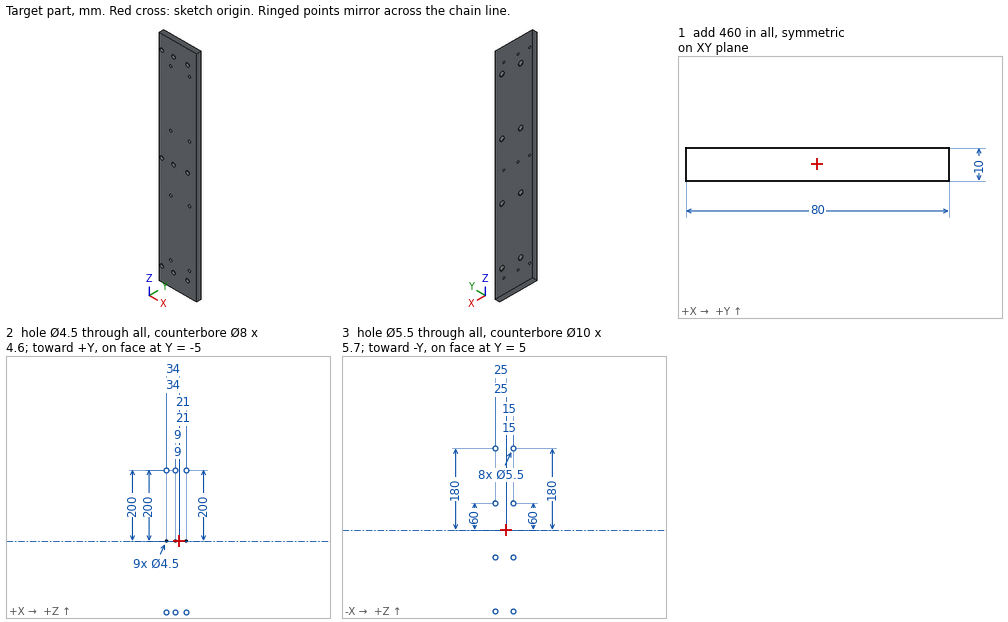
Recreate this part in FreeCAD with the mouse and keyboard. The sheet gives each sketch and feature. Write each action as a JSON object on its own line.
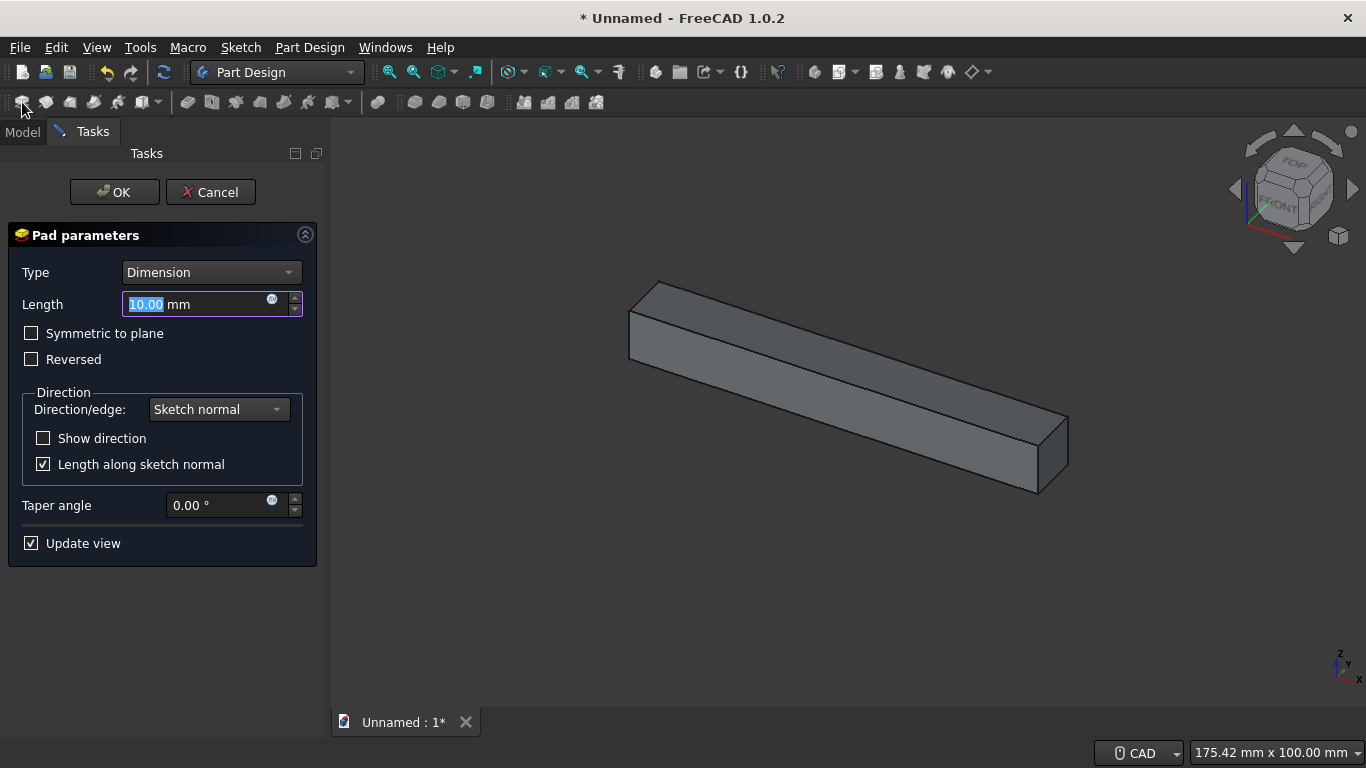
{"action": "type", "text": "460"}
{"action": "key", "text": "Tab"}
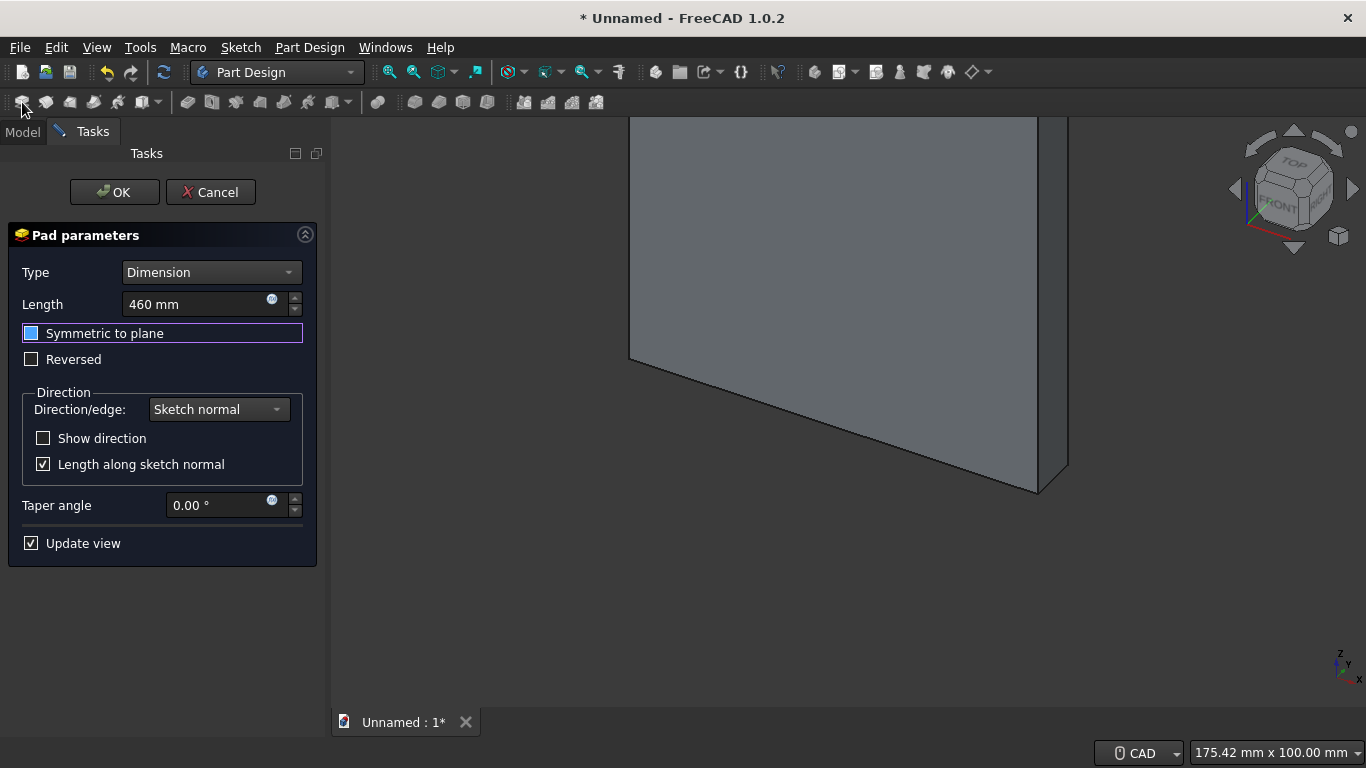
{"action": "left_click", "coordinate": [30, 333]}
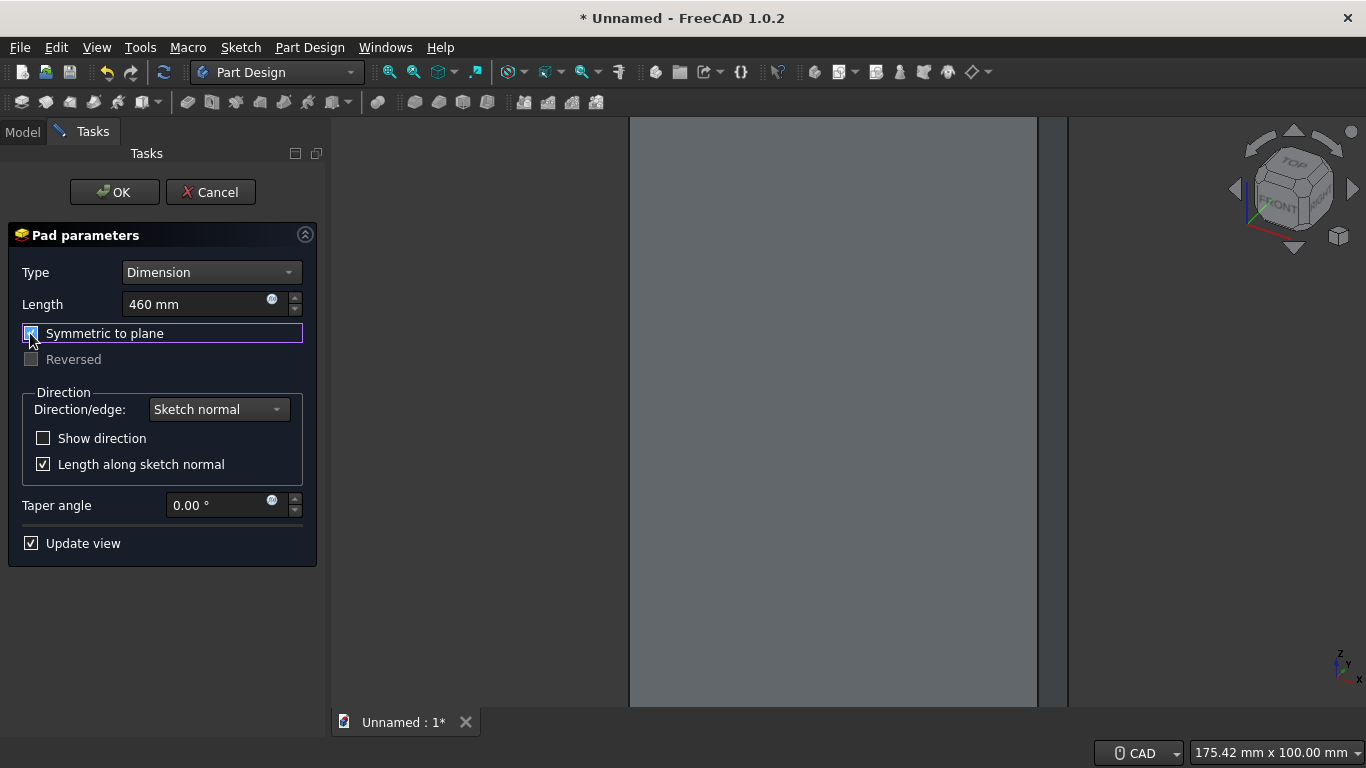
{"action": "left_click", "coordinate": [115, 192]}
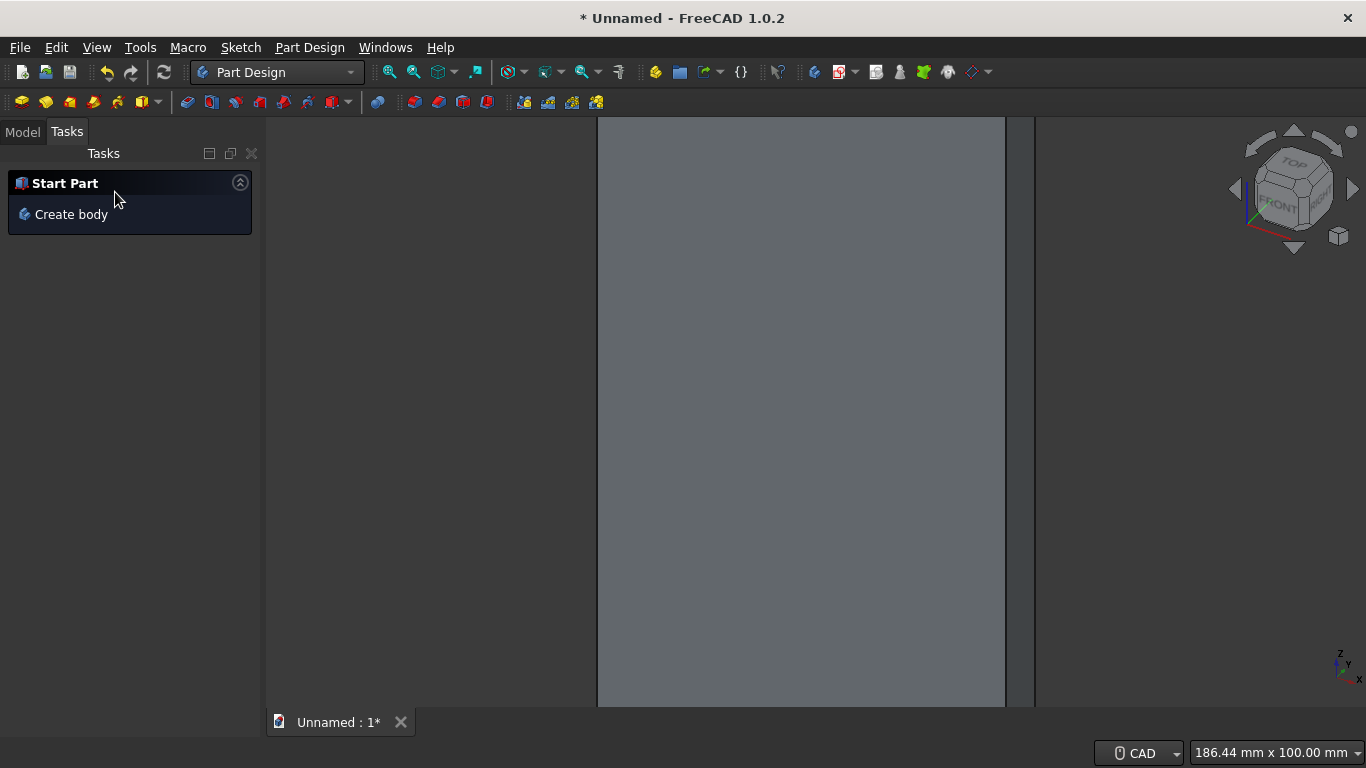
{"action": "left_click", "coordinate": [390, 72]}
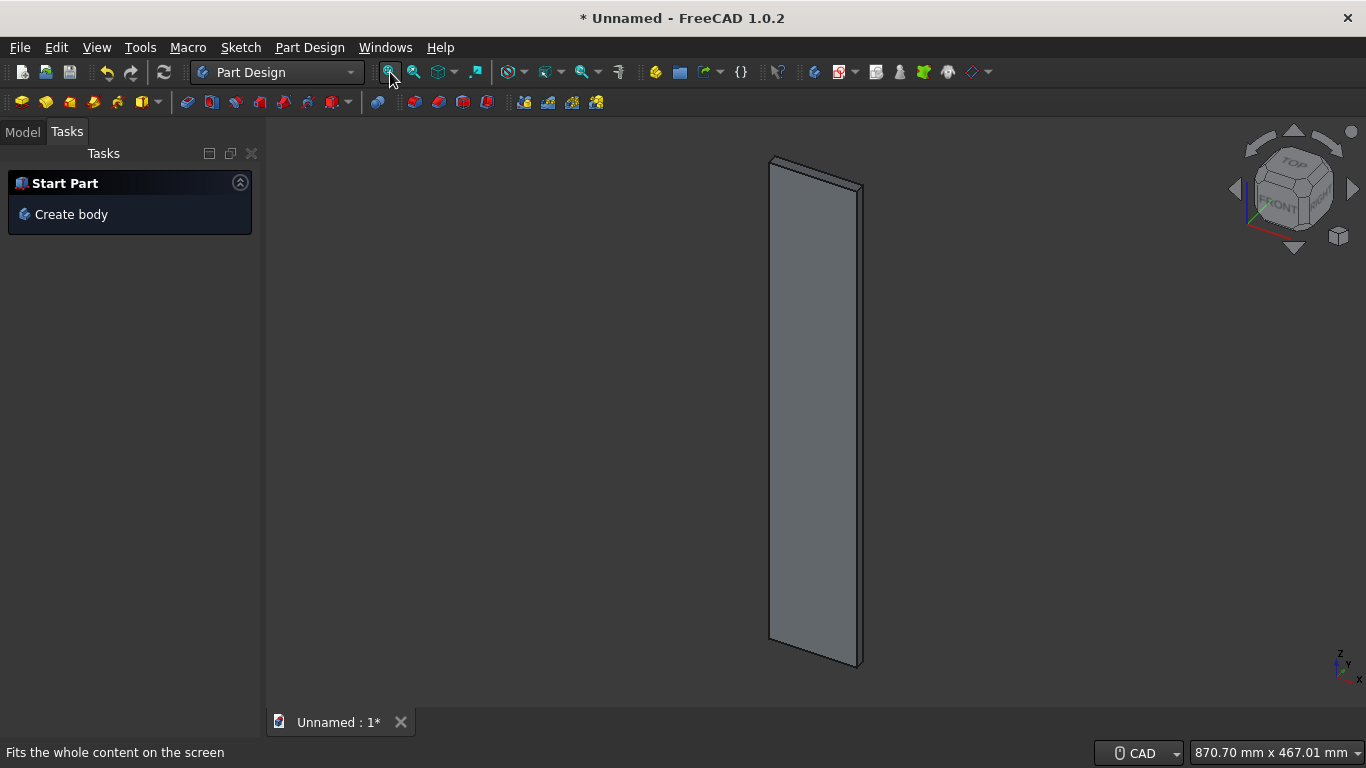
{"action": "left_click", "coordinate": [813, 278]}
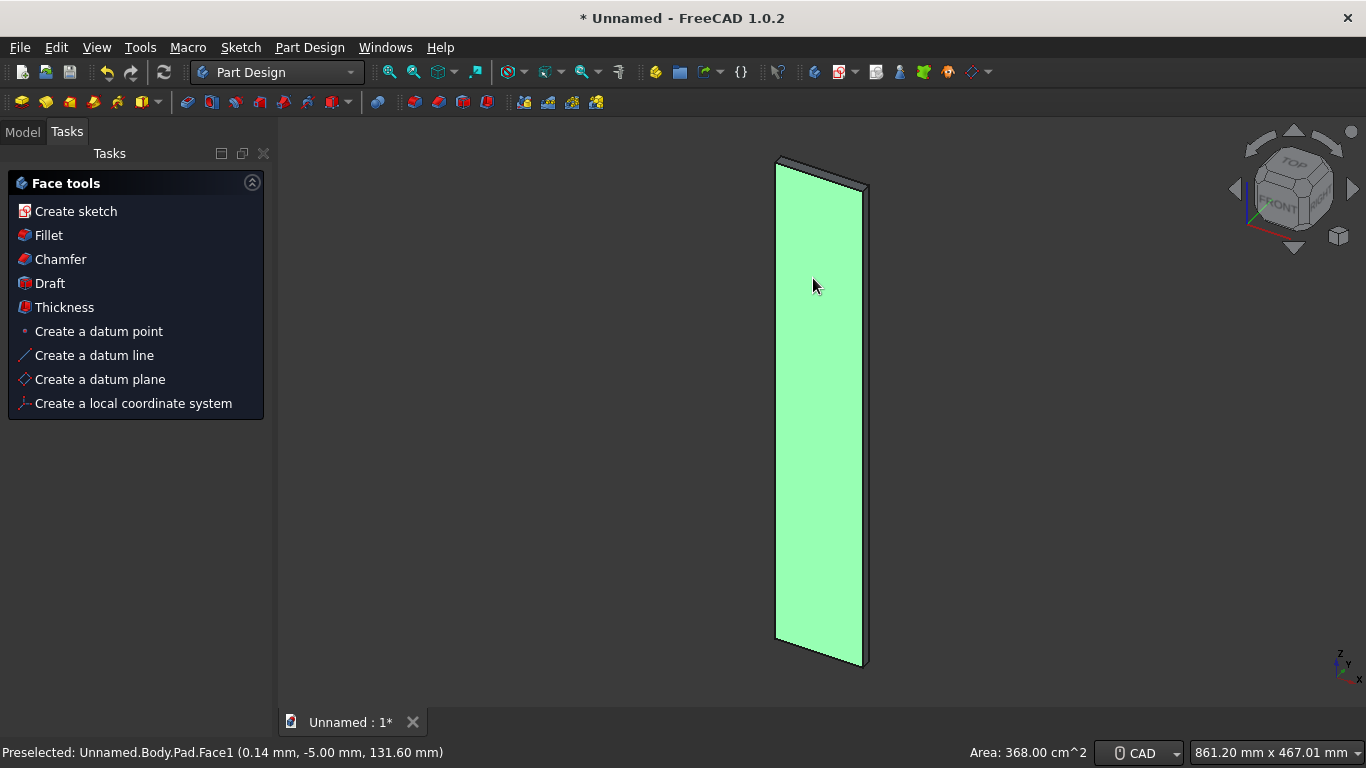
{"action": "left_click", "coordinate": [840, 72]}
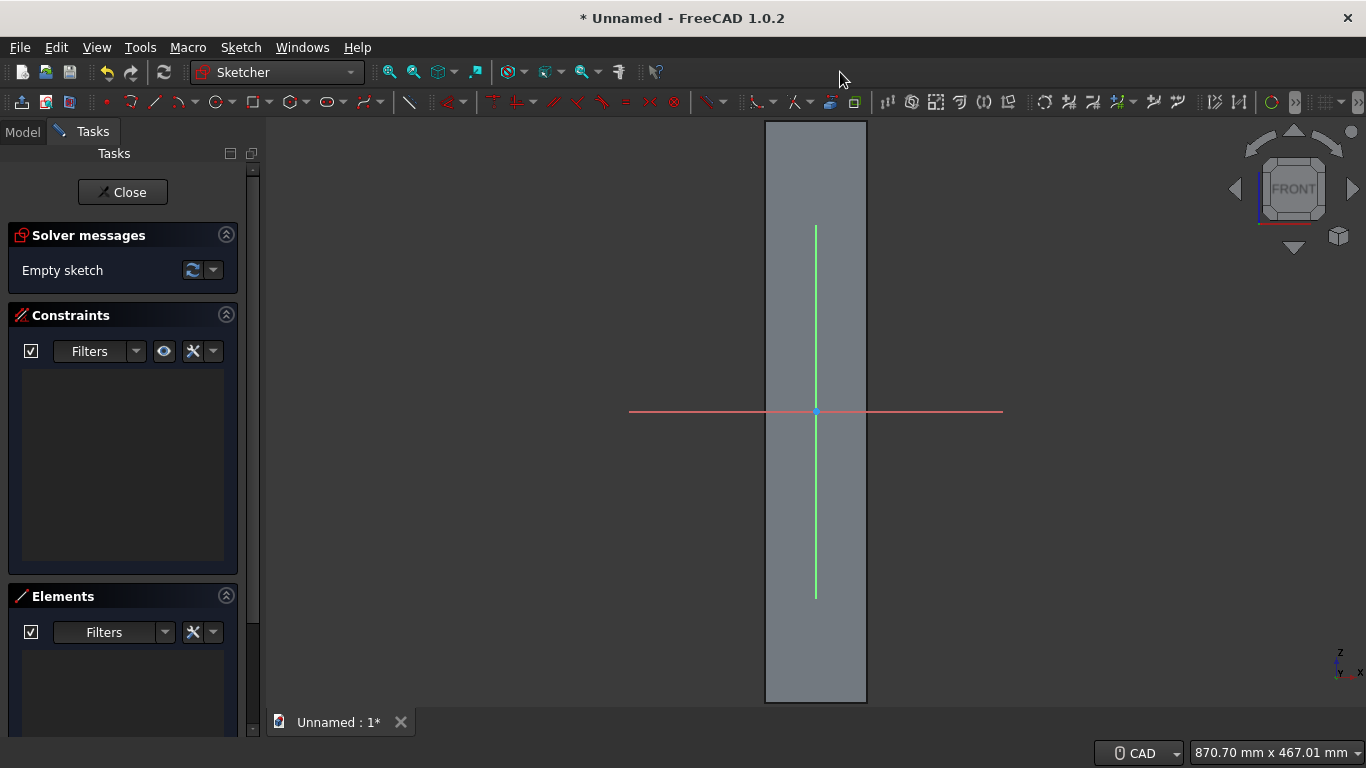
{"action": "scroll", "coordinate": [625, 412], "scroll_direction": "down", "scroll_amount": 2}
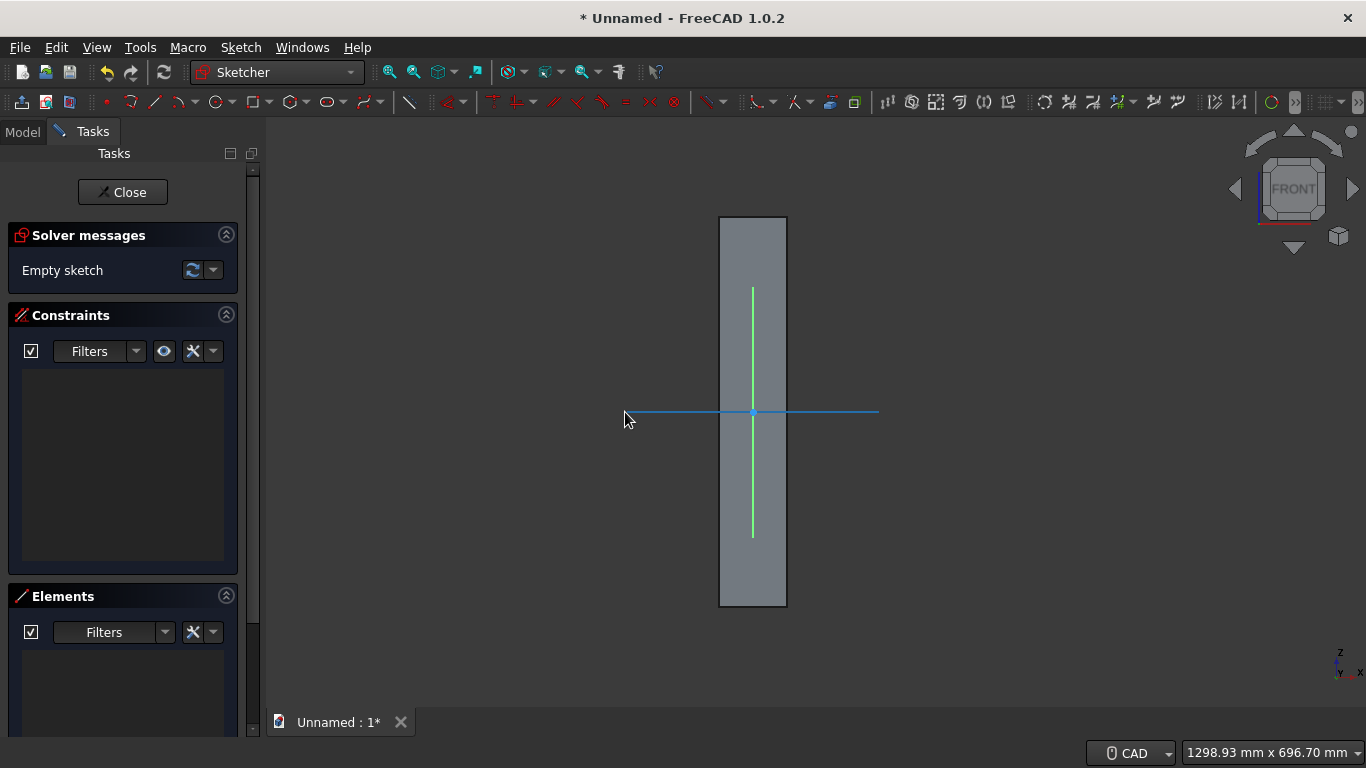
{"action": "key", "text": "g c"}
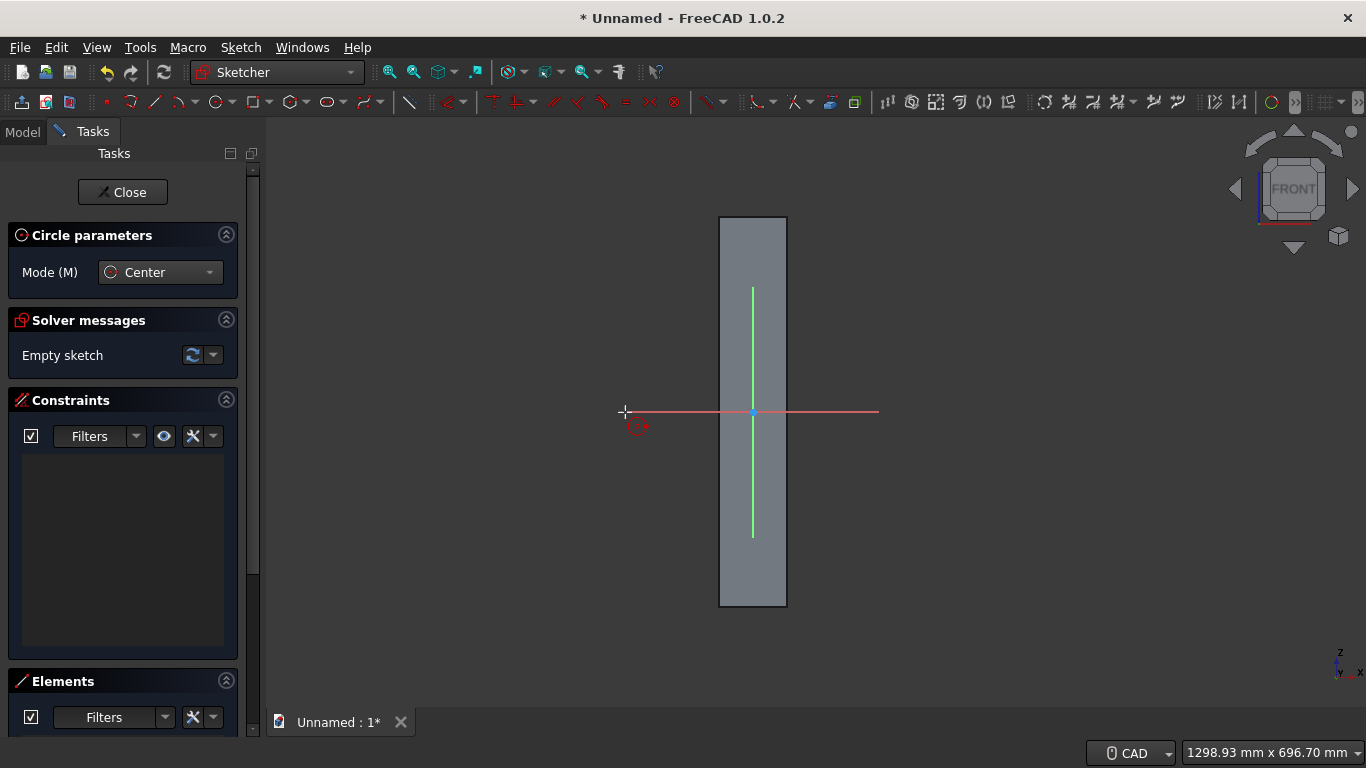
{"action": "scroll", "coordinate": [724, 243], "scroll_direction": "up", "scroll_amount": 13}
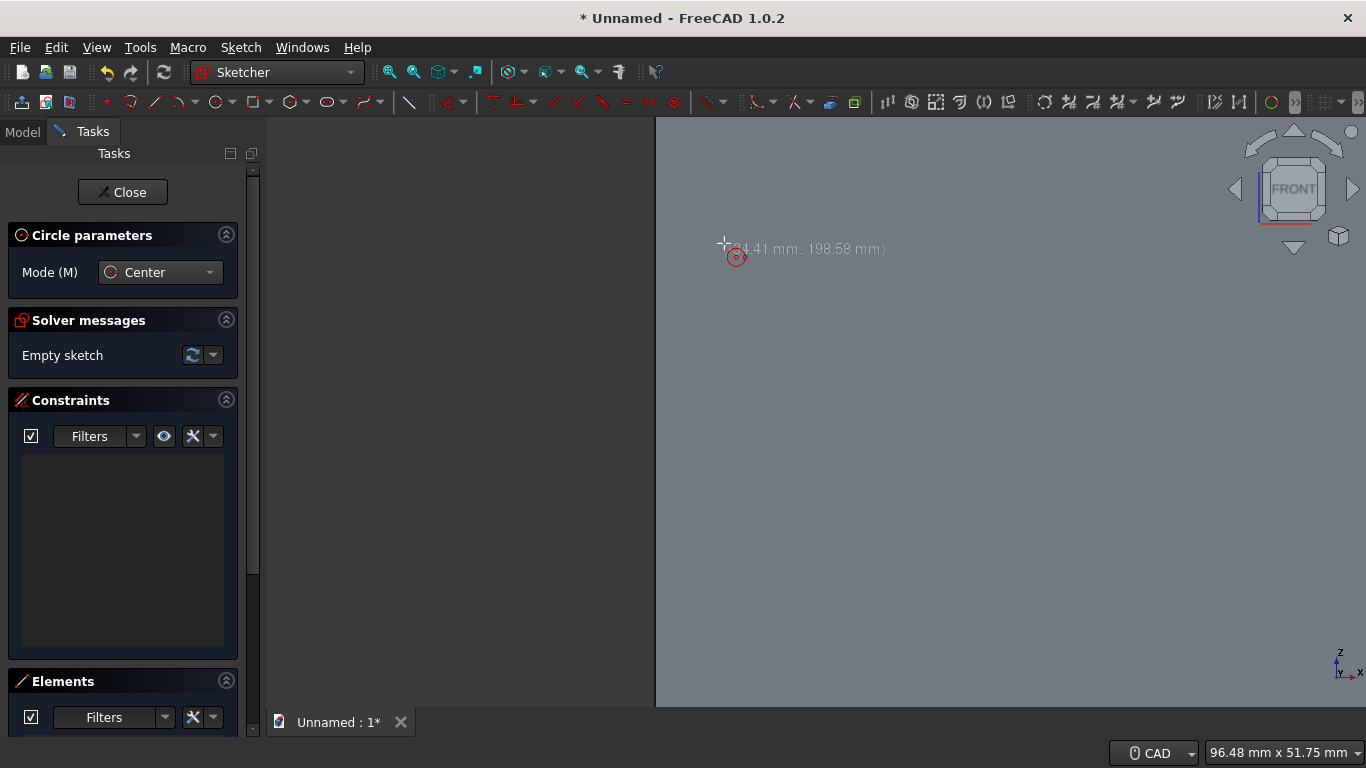
{"action": "scroll", "coordinate": [724, 243], "scroll_direction": "down", "scroll_amount": 13}